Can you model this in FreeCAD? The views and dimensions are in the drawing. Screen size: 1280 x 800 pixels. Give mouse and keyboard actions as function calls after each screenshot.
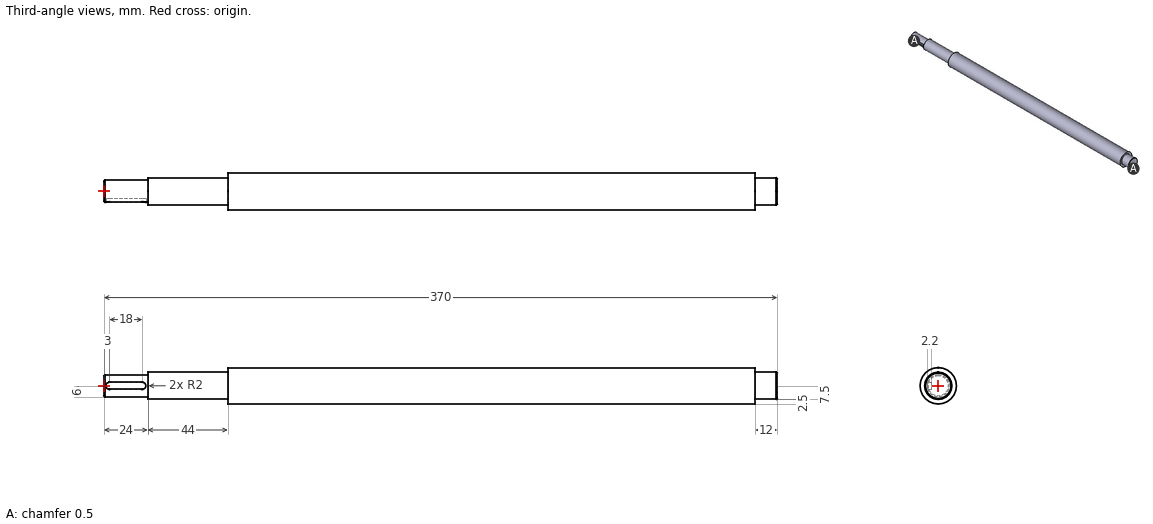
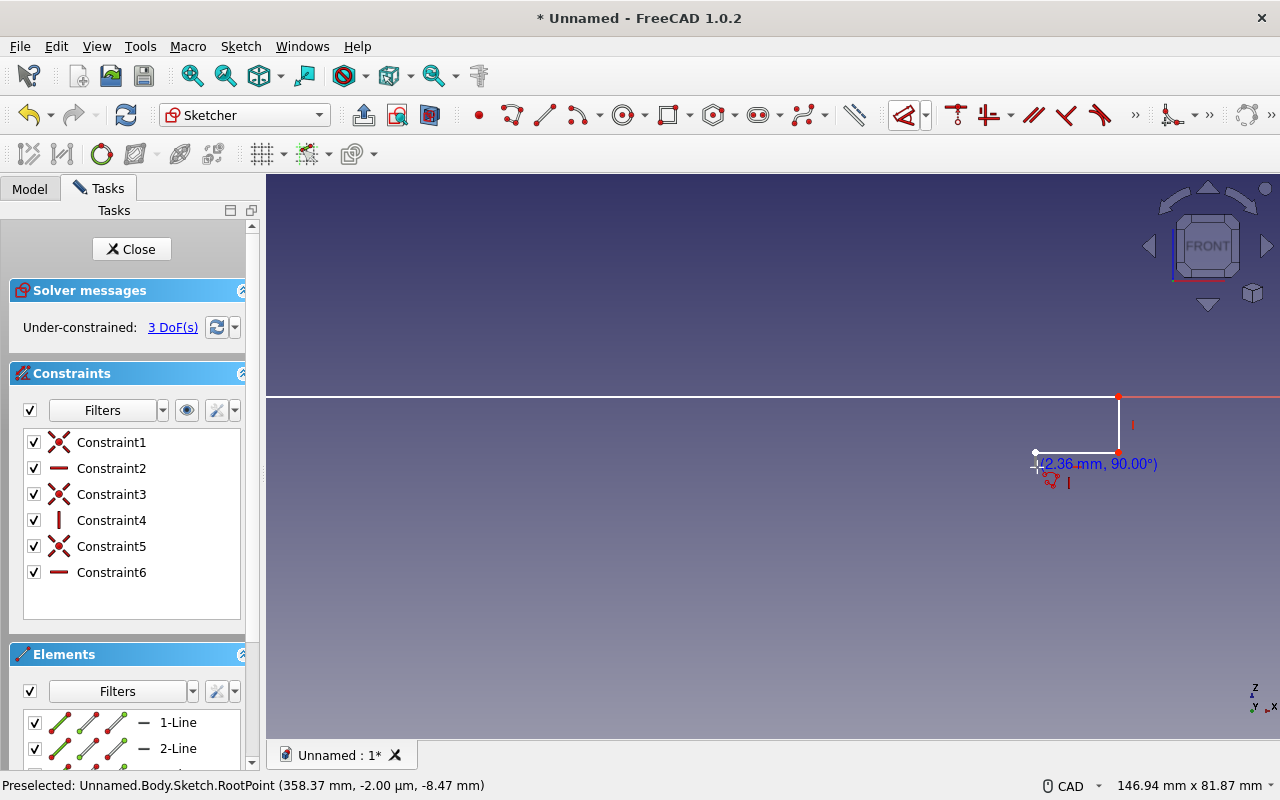
click(1036, 466)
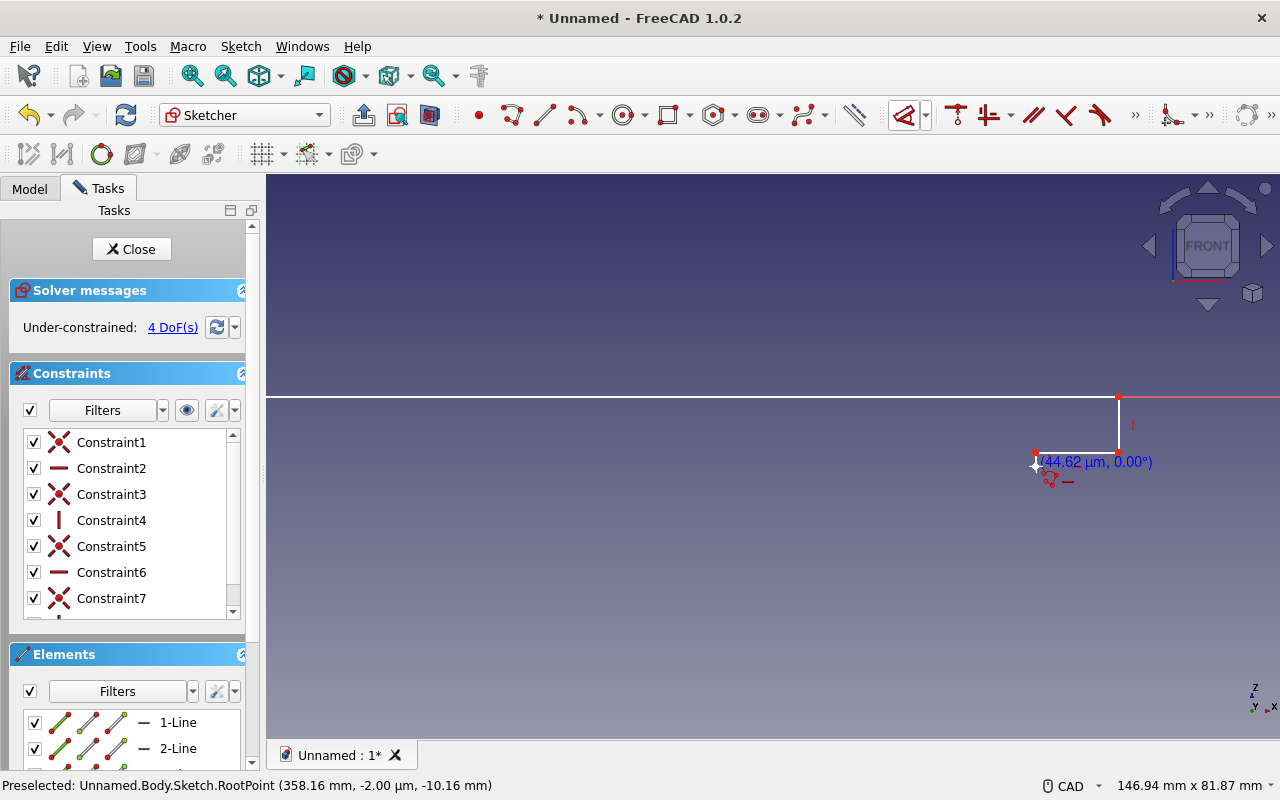
scroll(987, 465, down, 7)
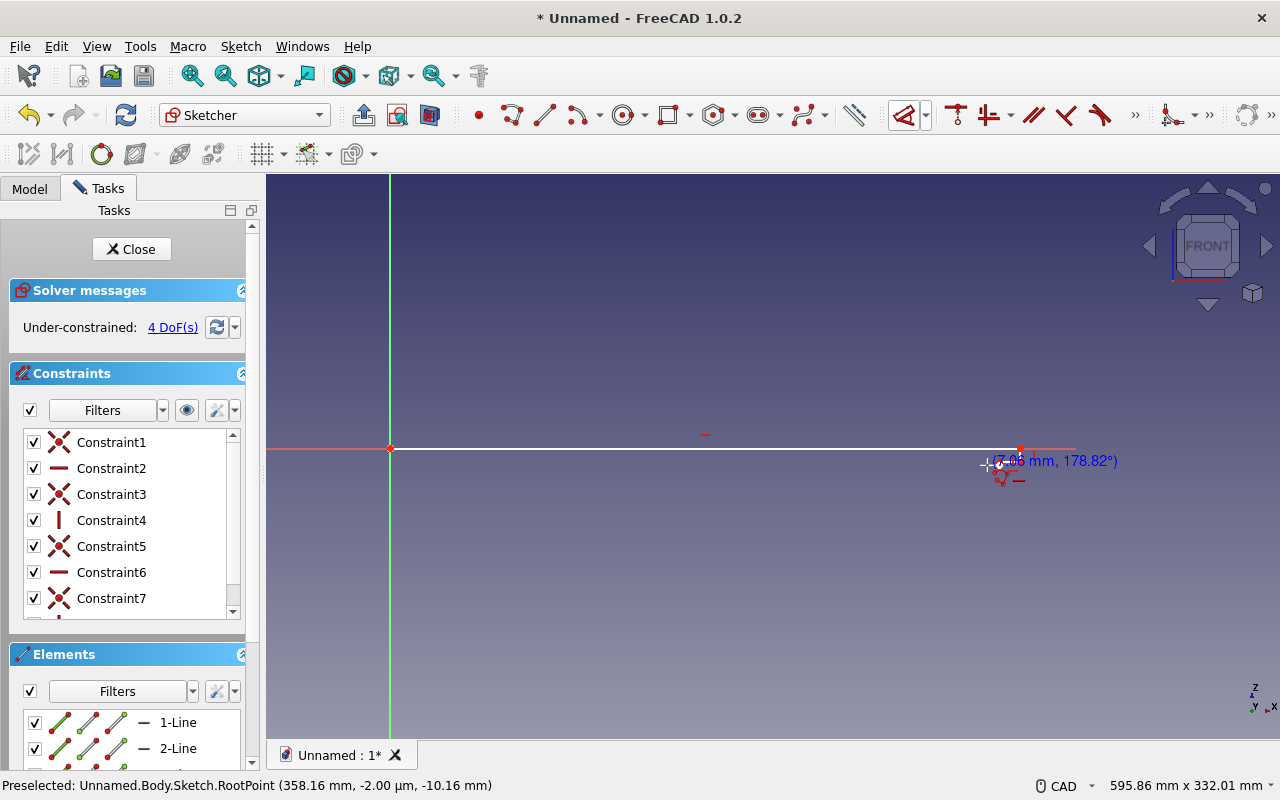
click(506, 466)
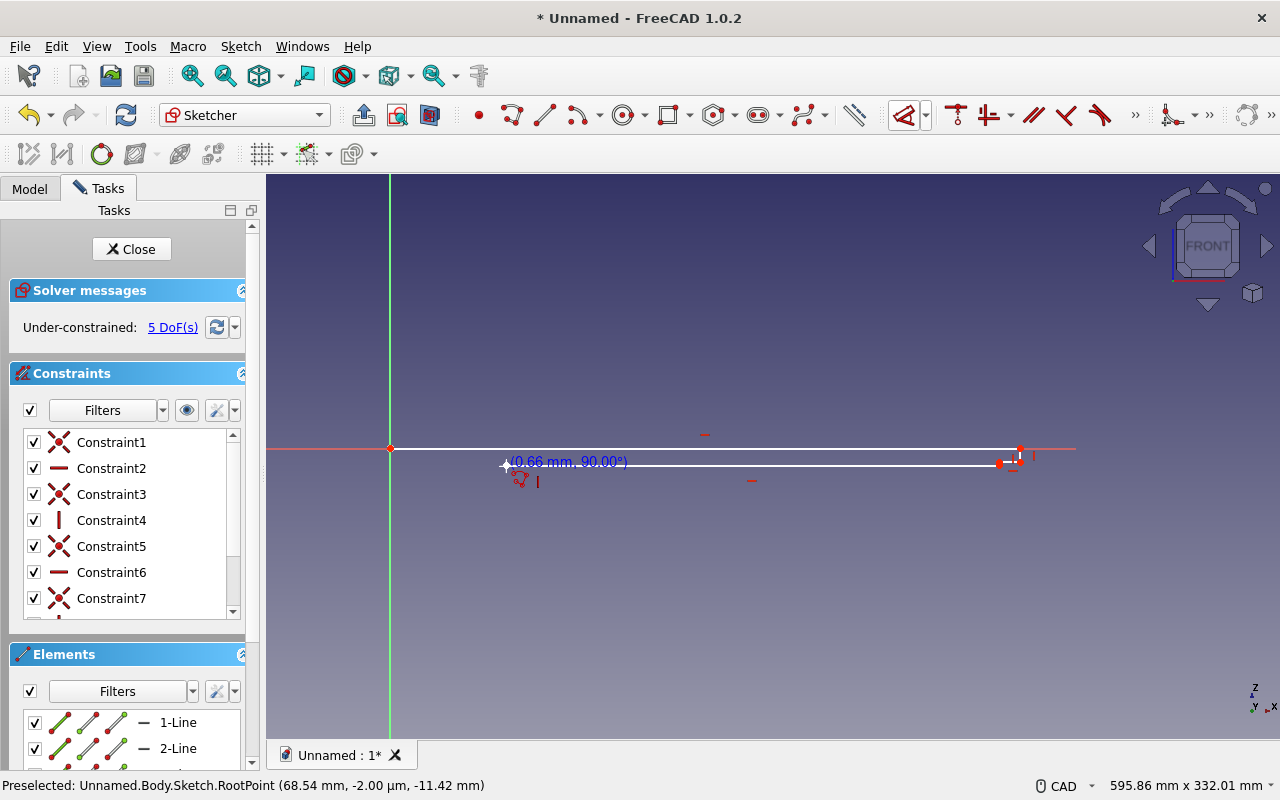
scroll(506, 461, up, 7)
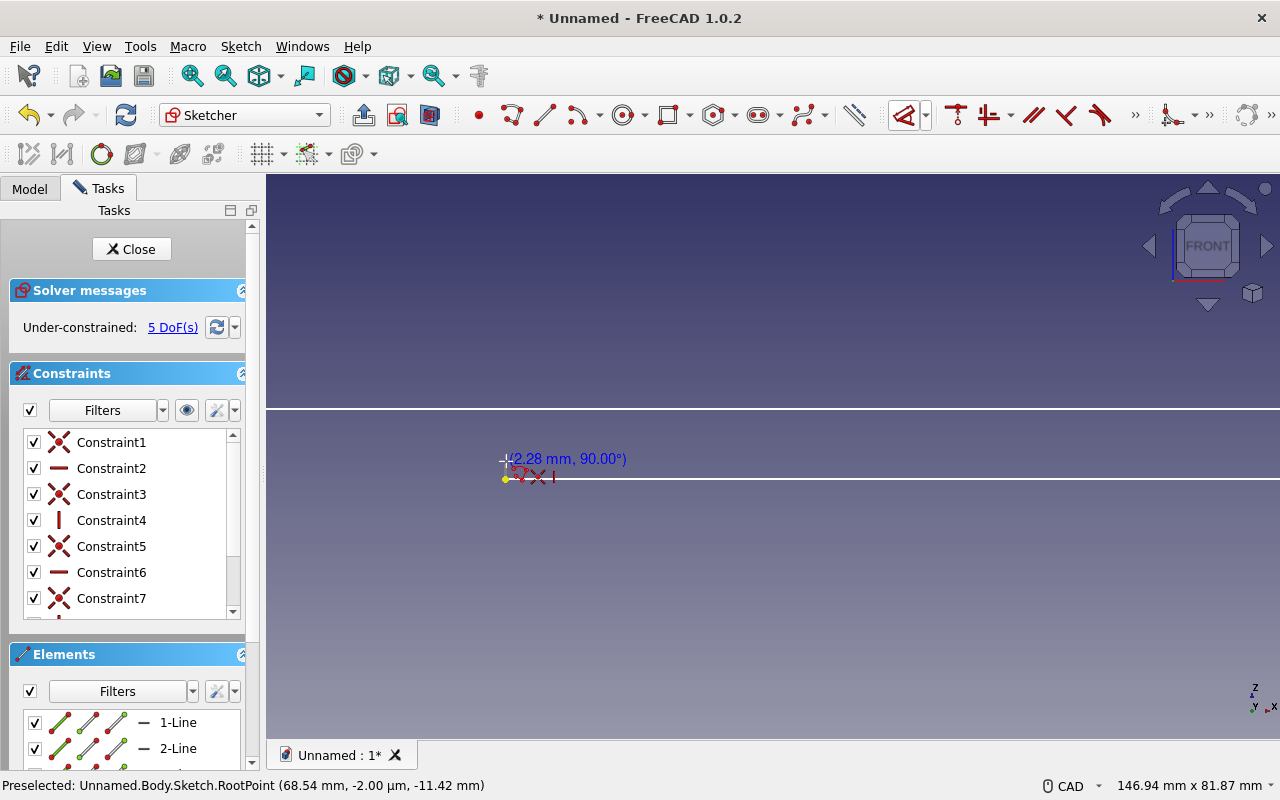
click(505, 461)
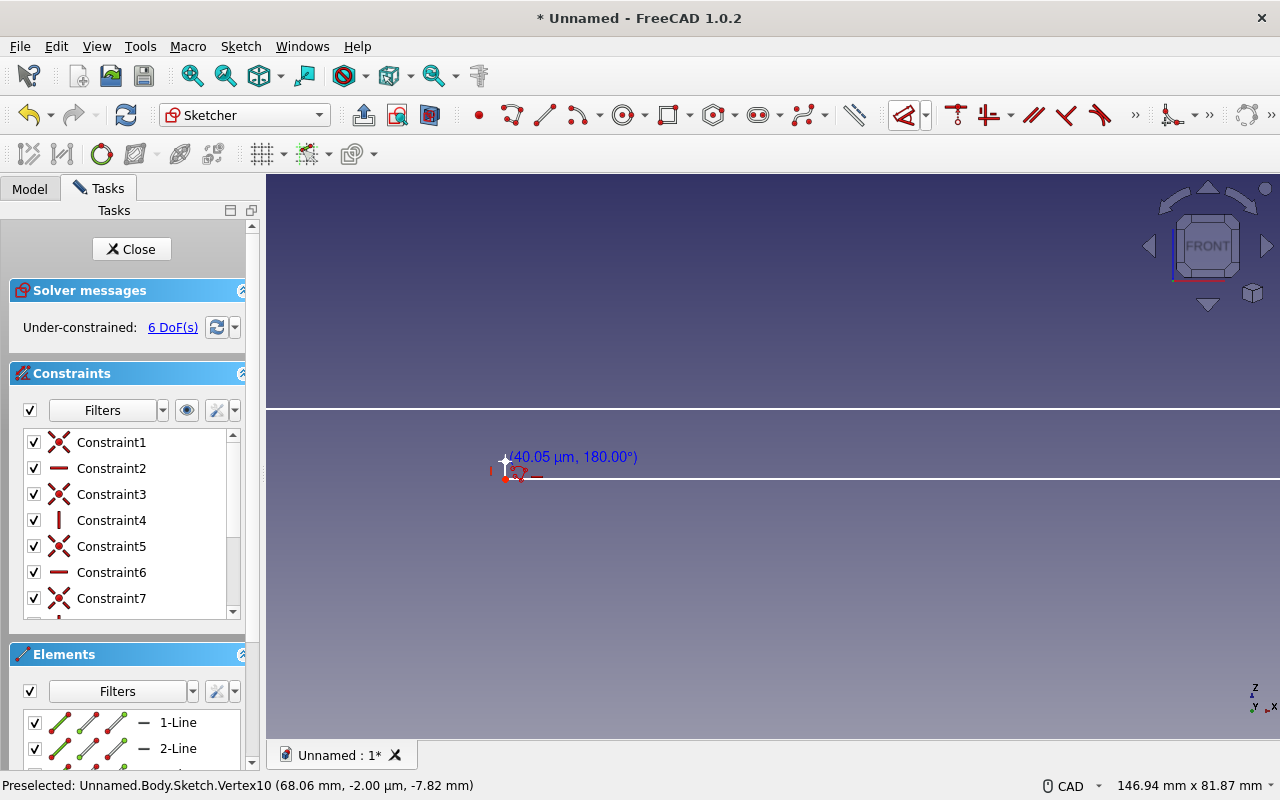
scroll(505, 461, down, 7)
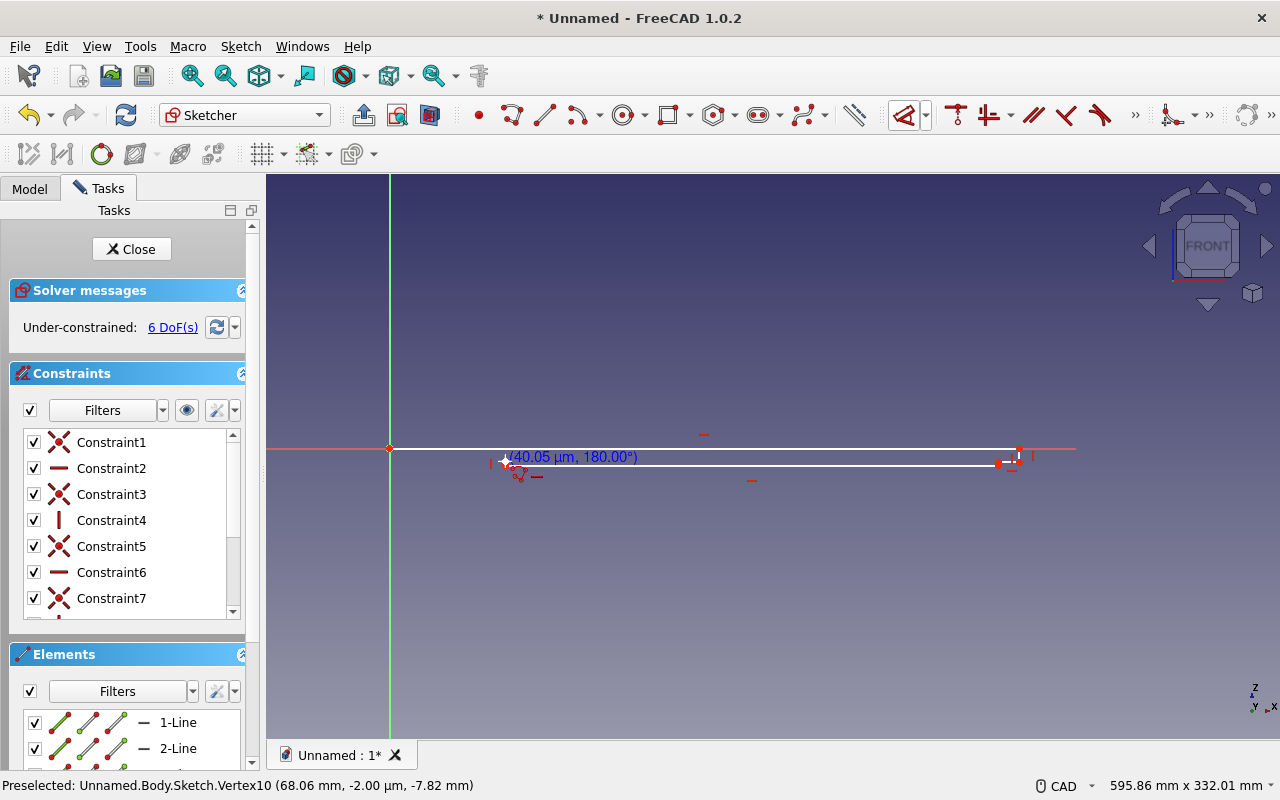
scroll(430, 461, up, 2)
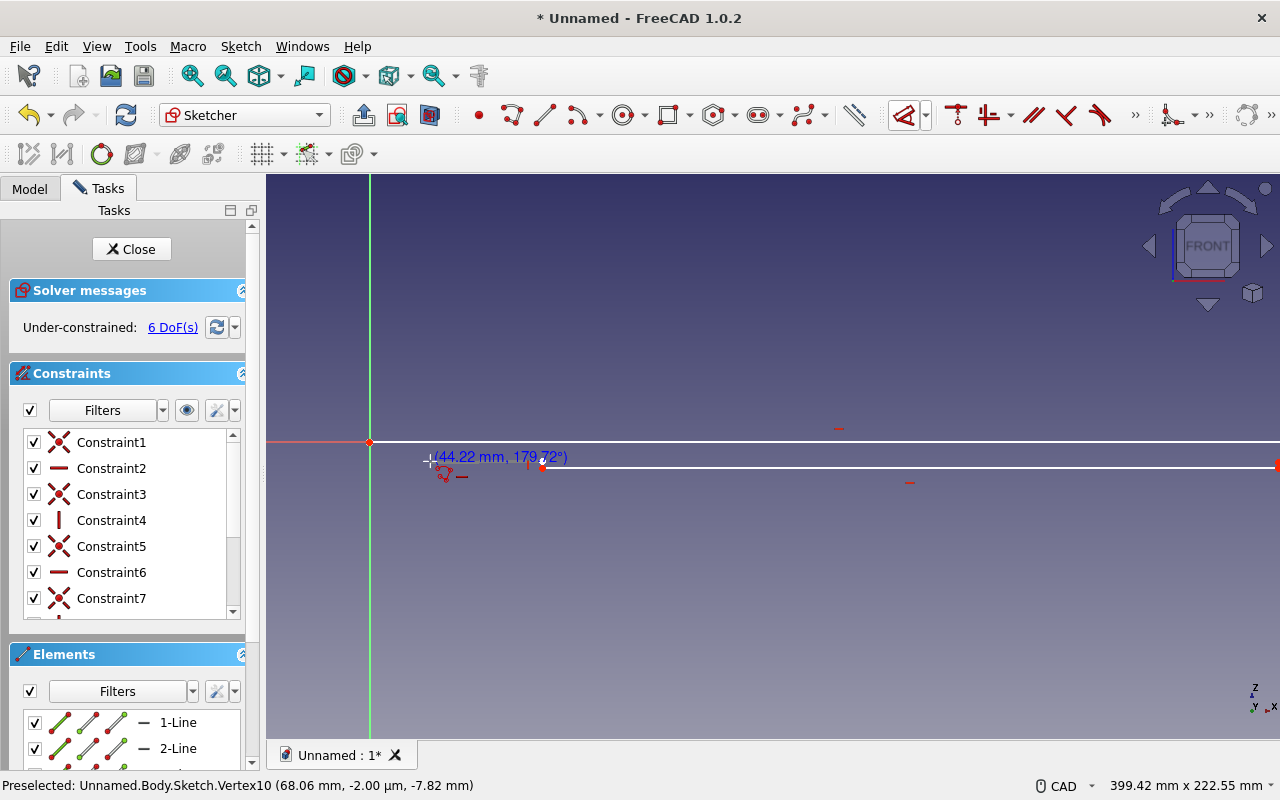
click(431, 461)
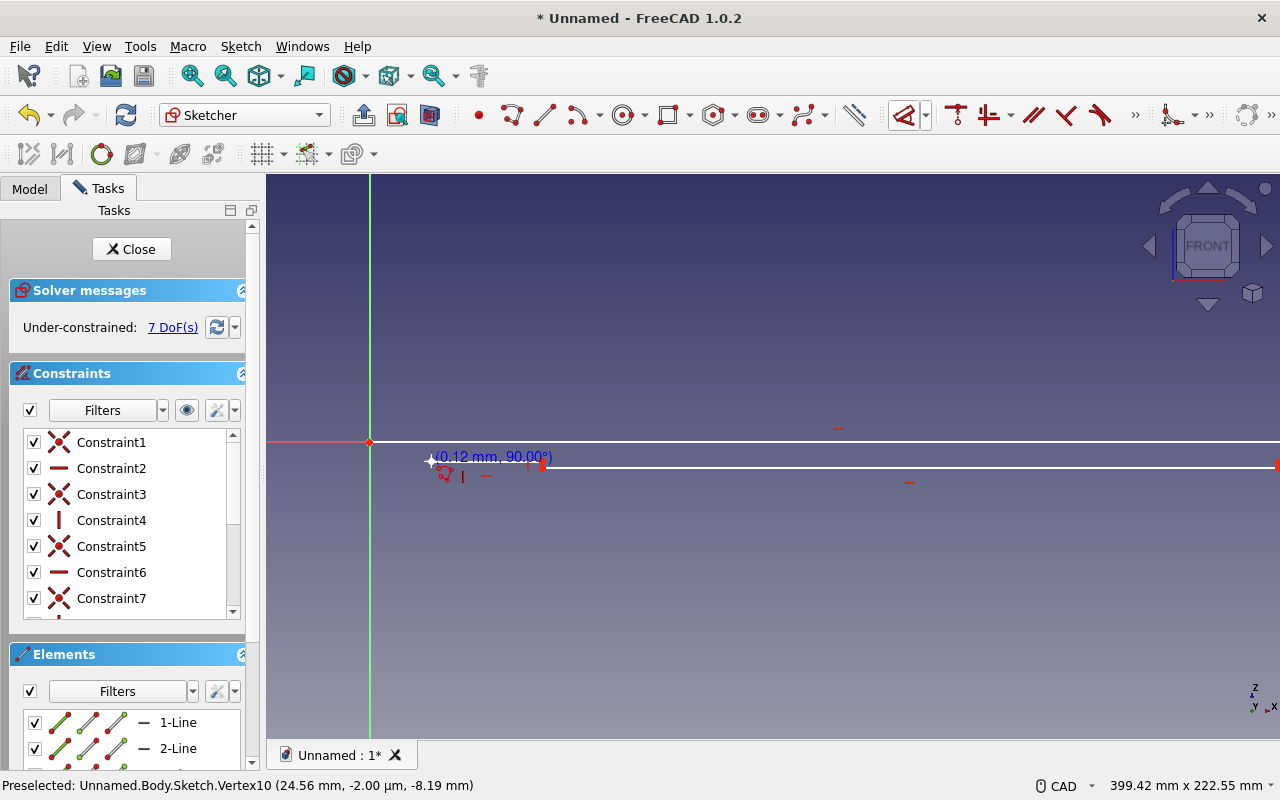
scroll(431, 457, up, 8)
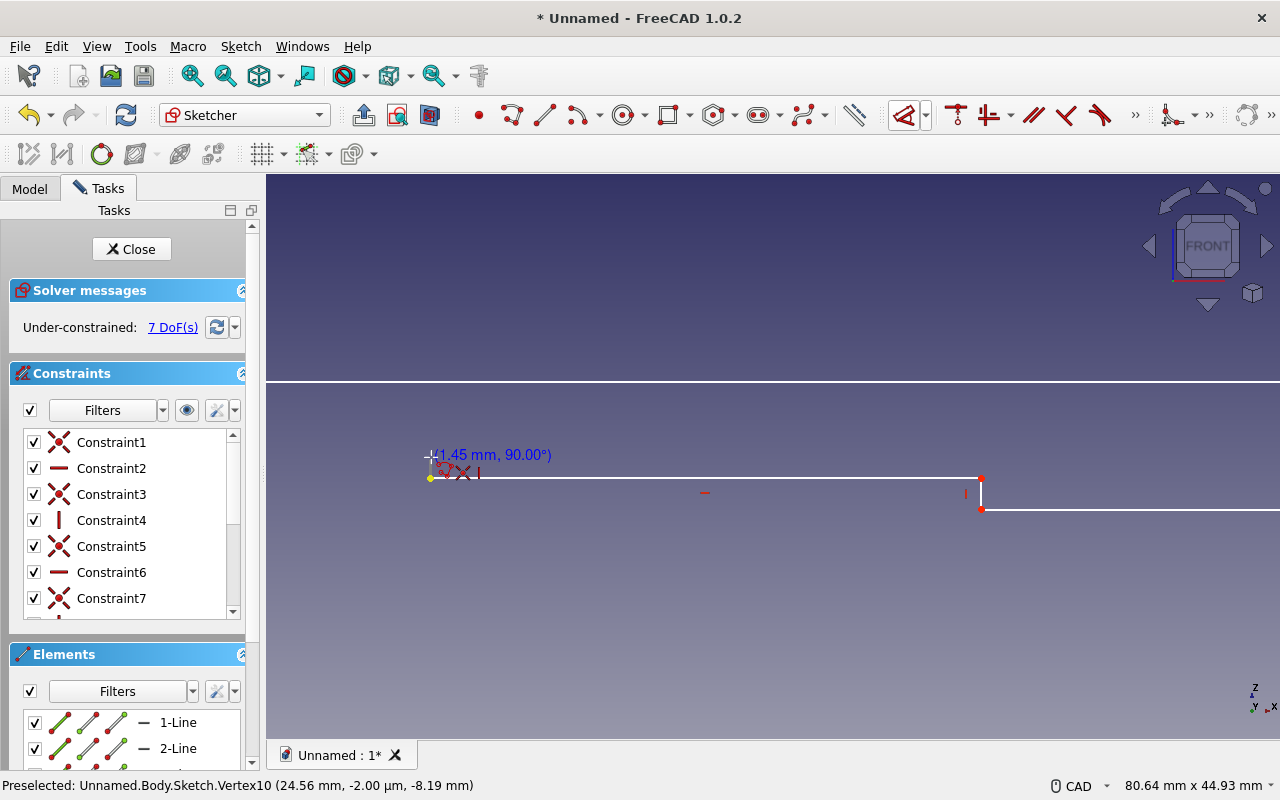
click(430, 457)